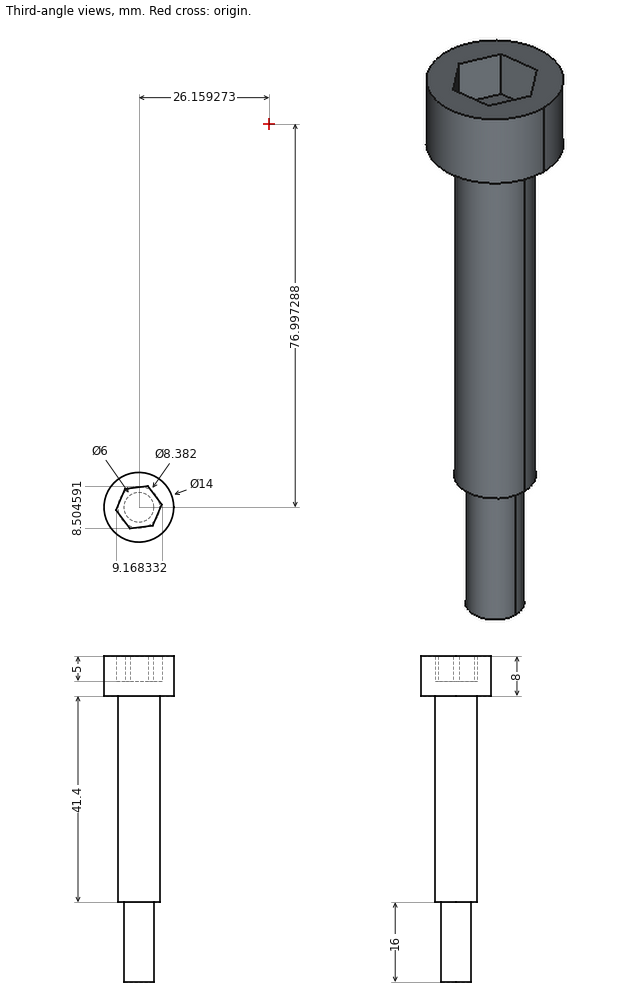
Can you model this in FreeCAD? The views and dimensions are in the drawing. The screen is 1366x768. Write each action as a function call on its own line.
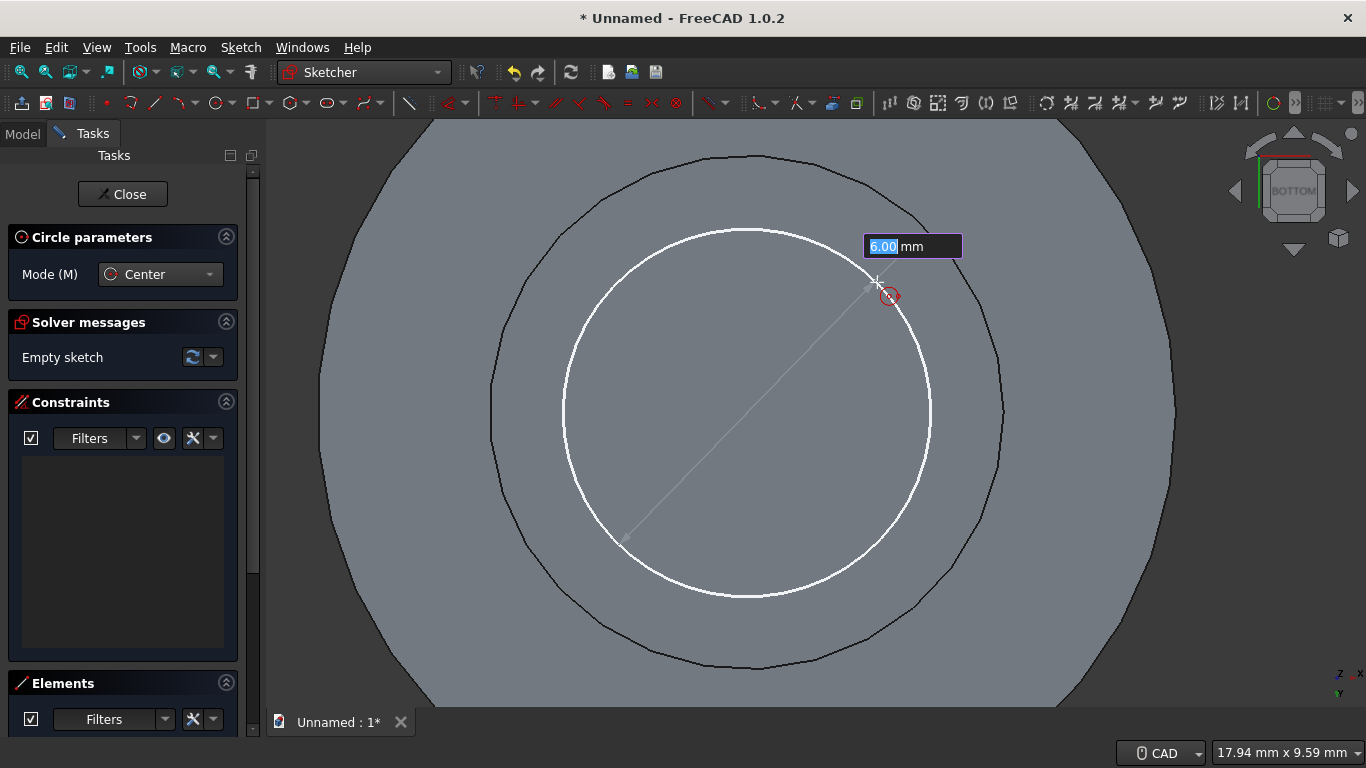
text(6)
key(Return)
key(Escape)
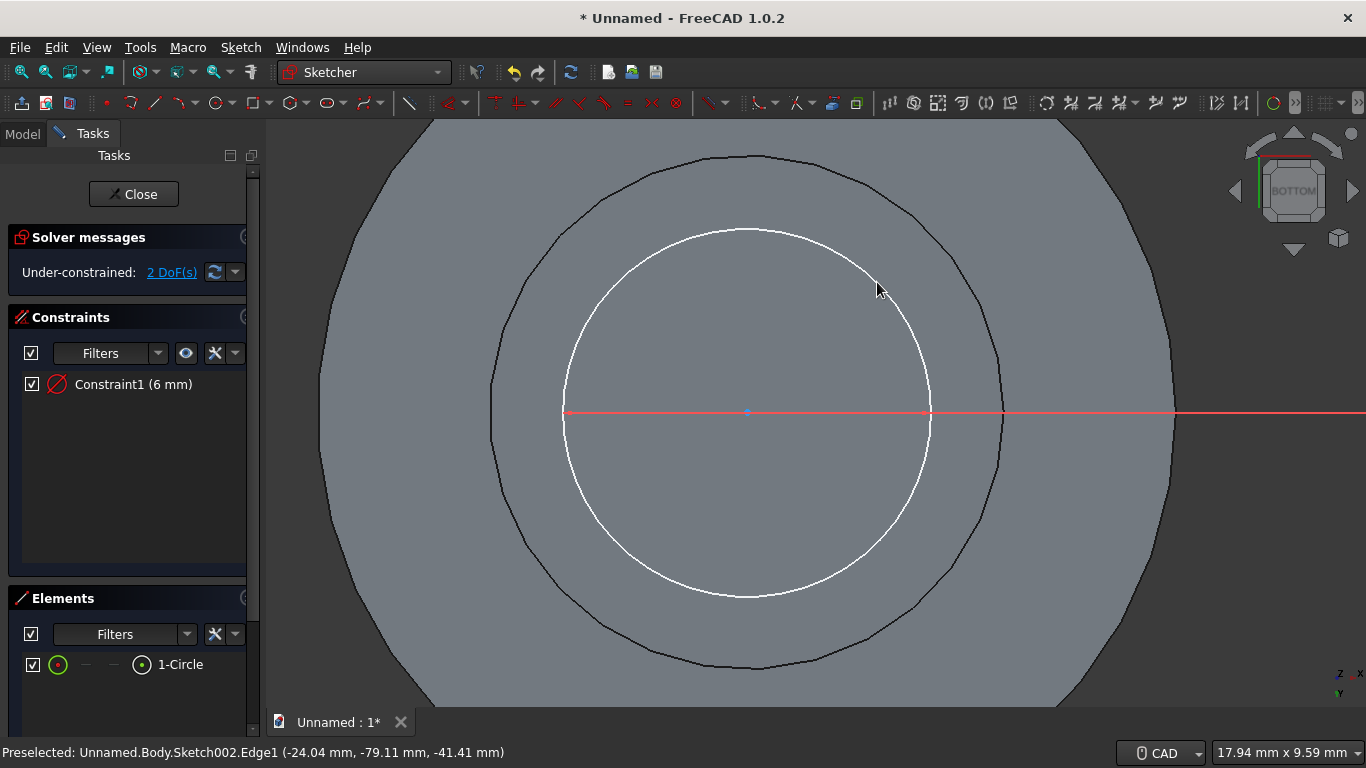
click(448, 104)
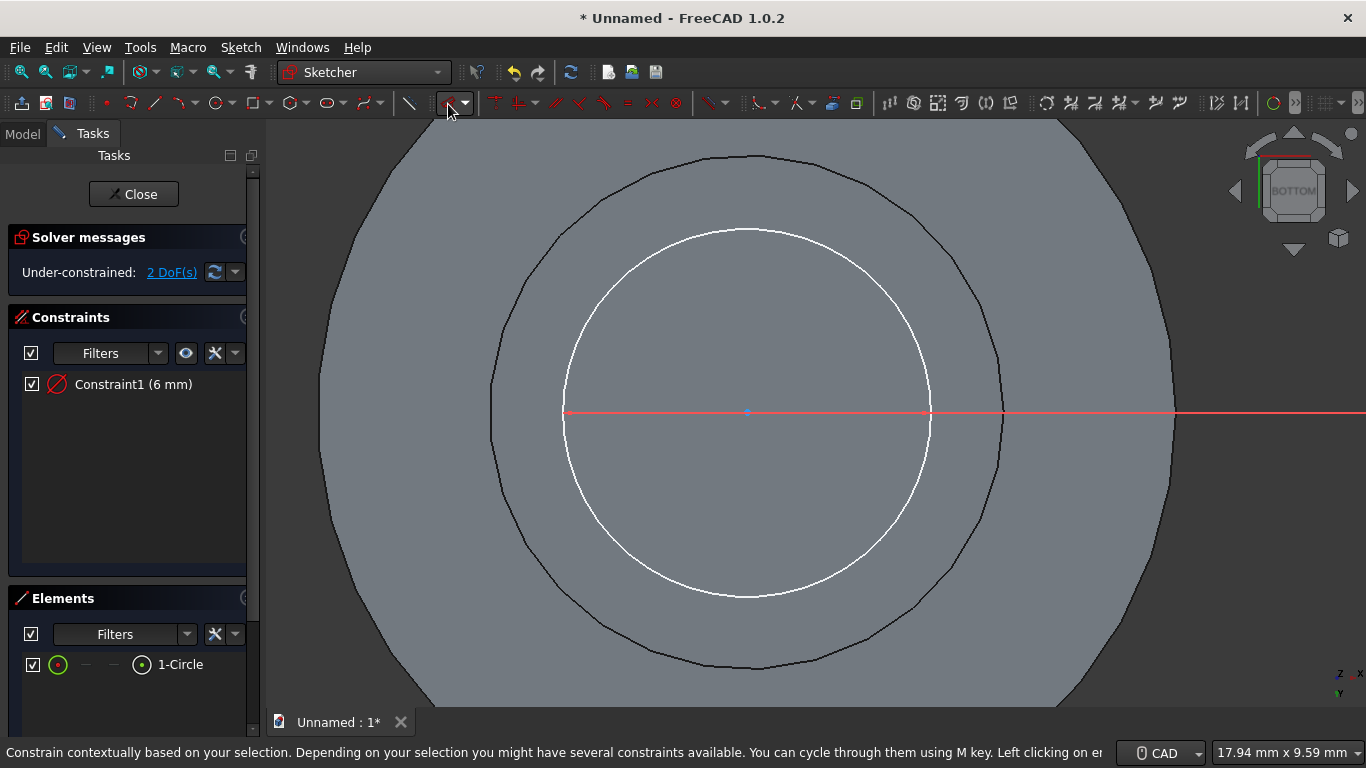
click(747, 413)
click(974, 379)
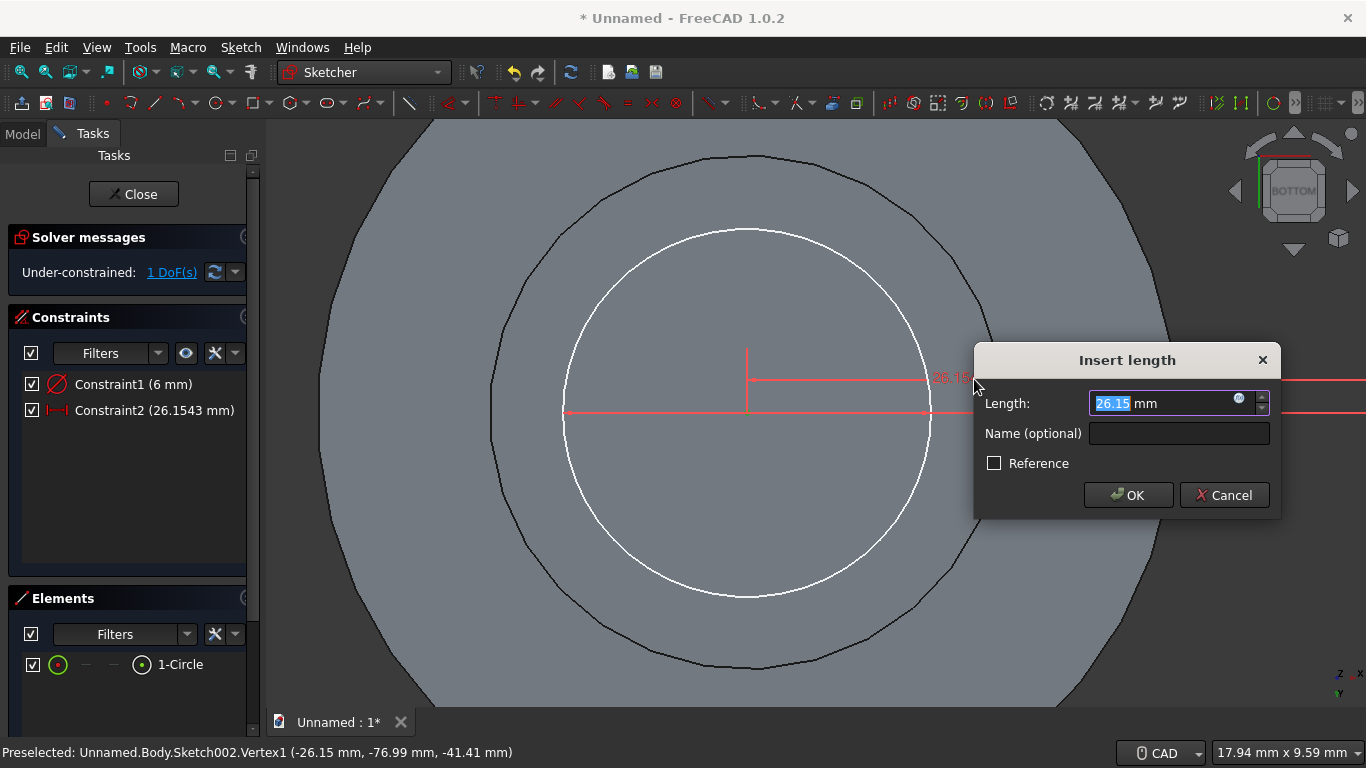
text(26.159273)
key(Return)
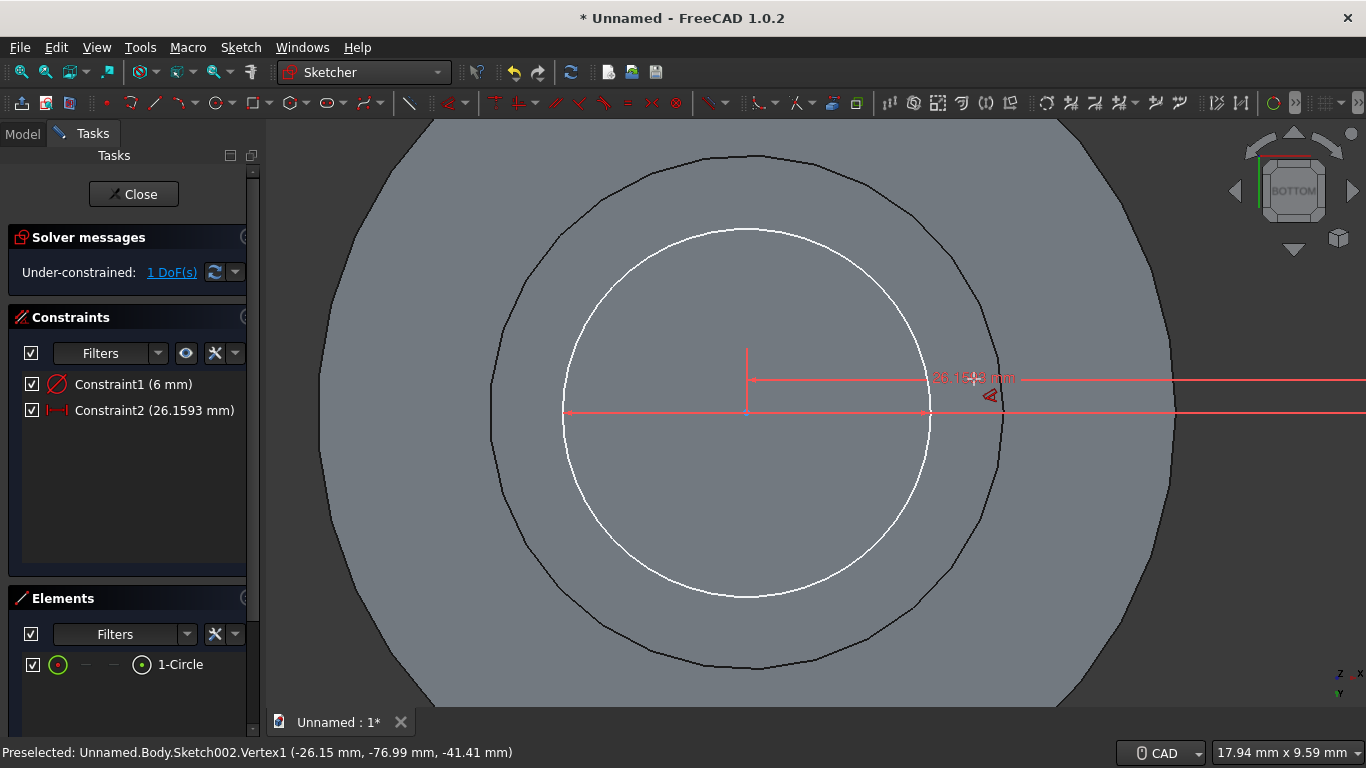
click(747, 413)
click(713, 546)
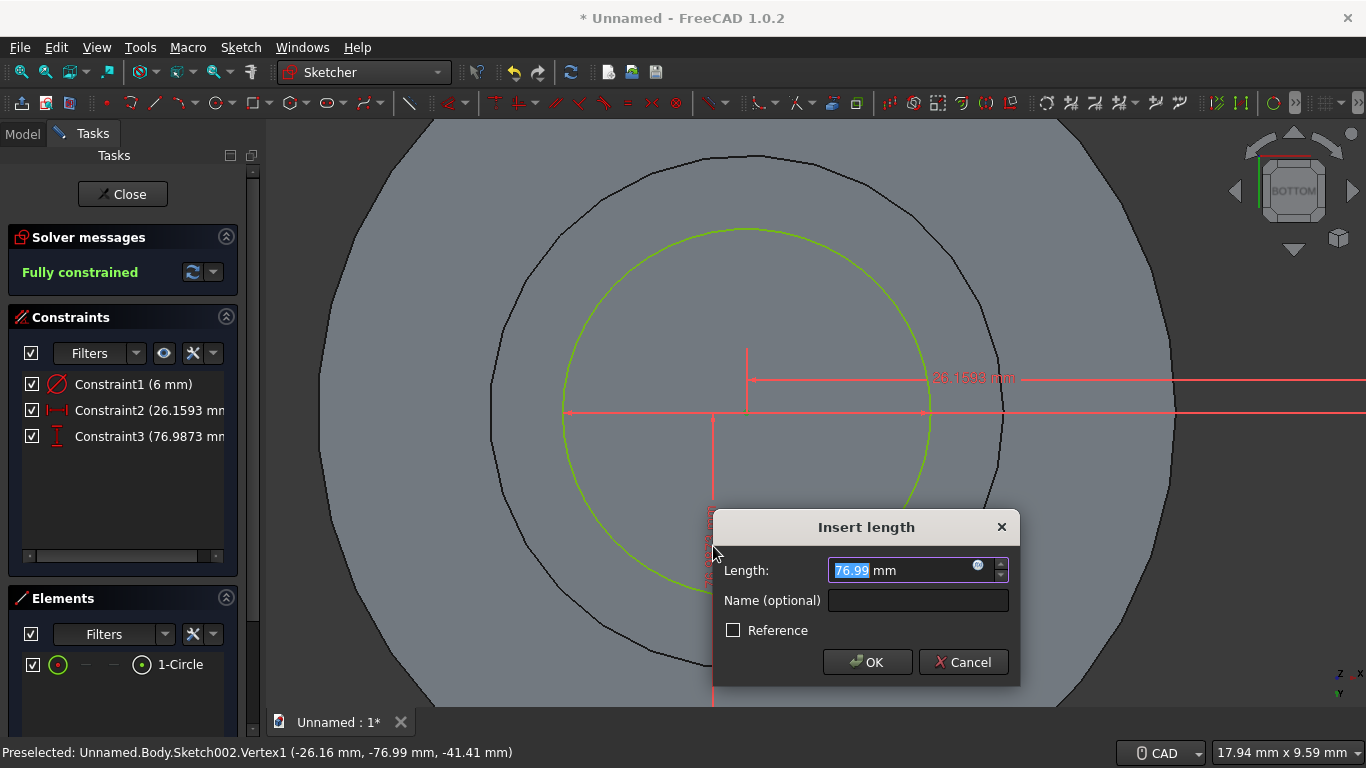
text(76.997288)
key(Return)
key(Escape)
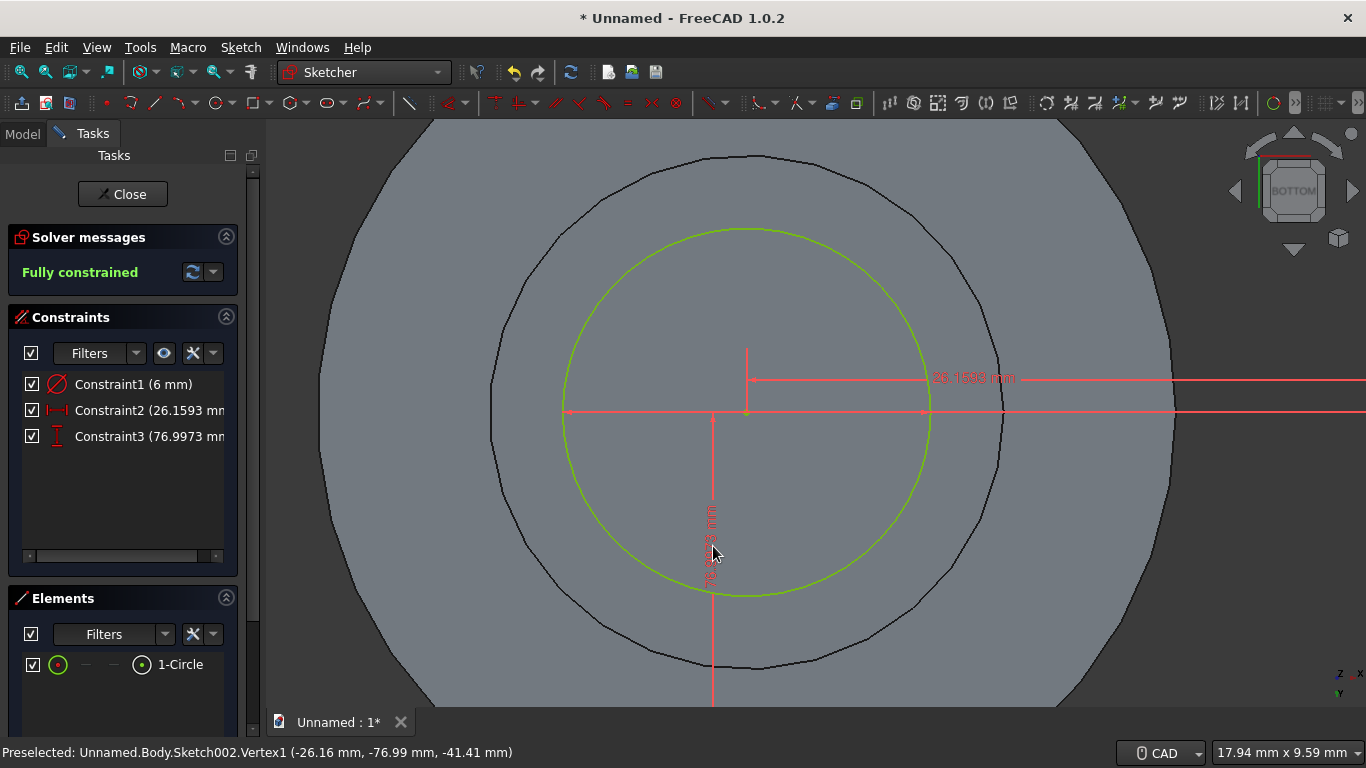
click(123, 194)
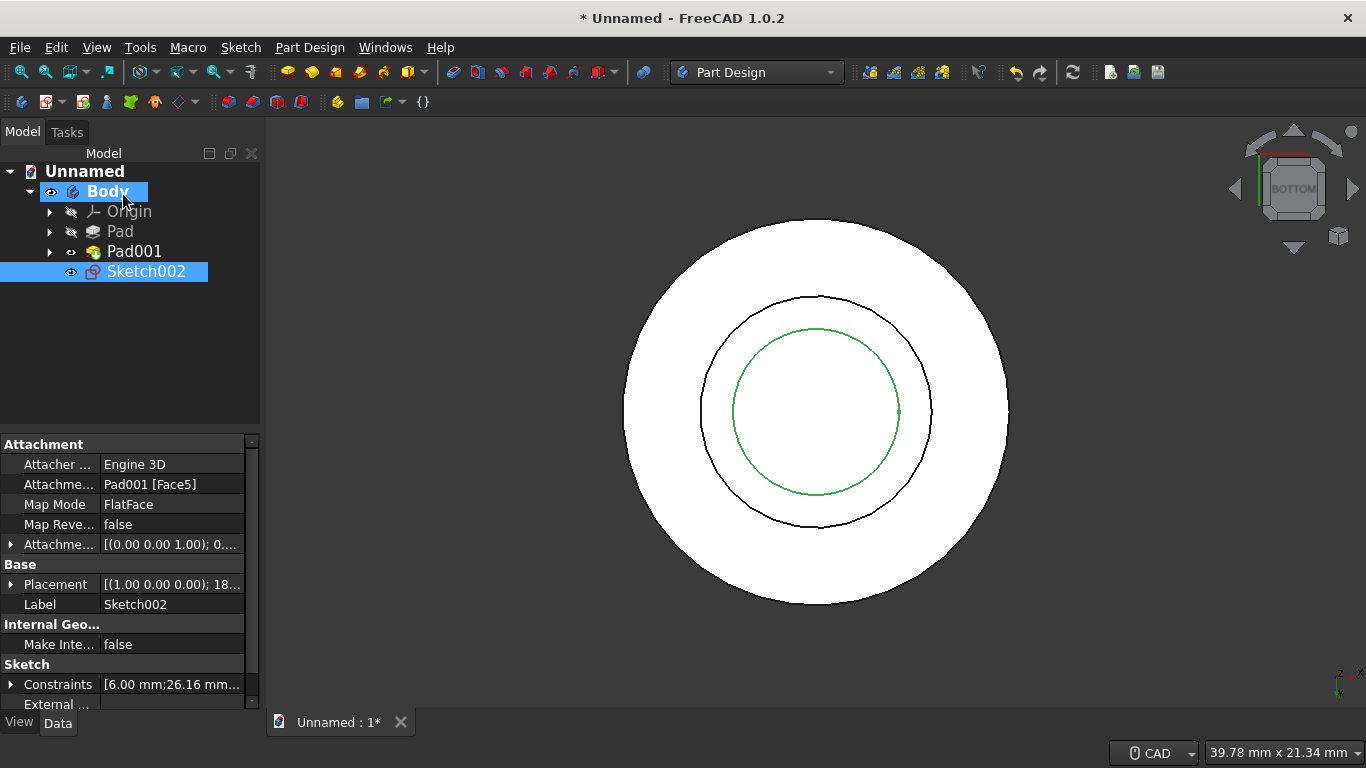
click(288, 72)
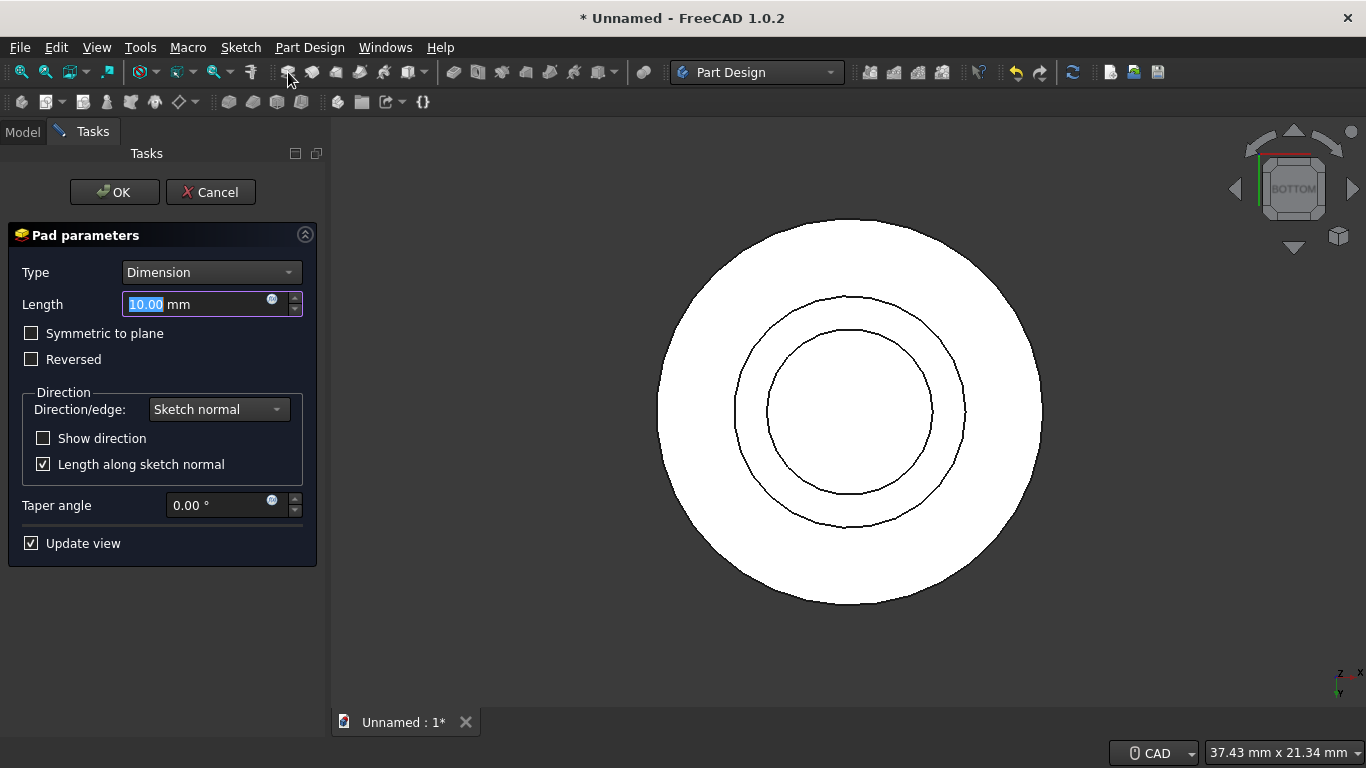
text(16)
key(Tab)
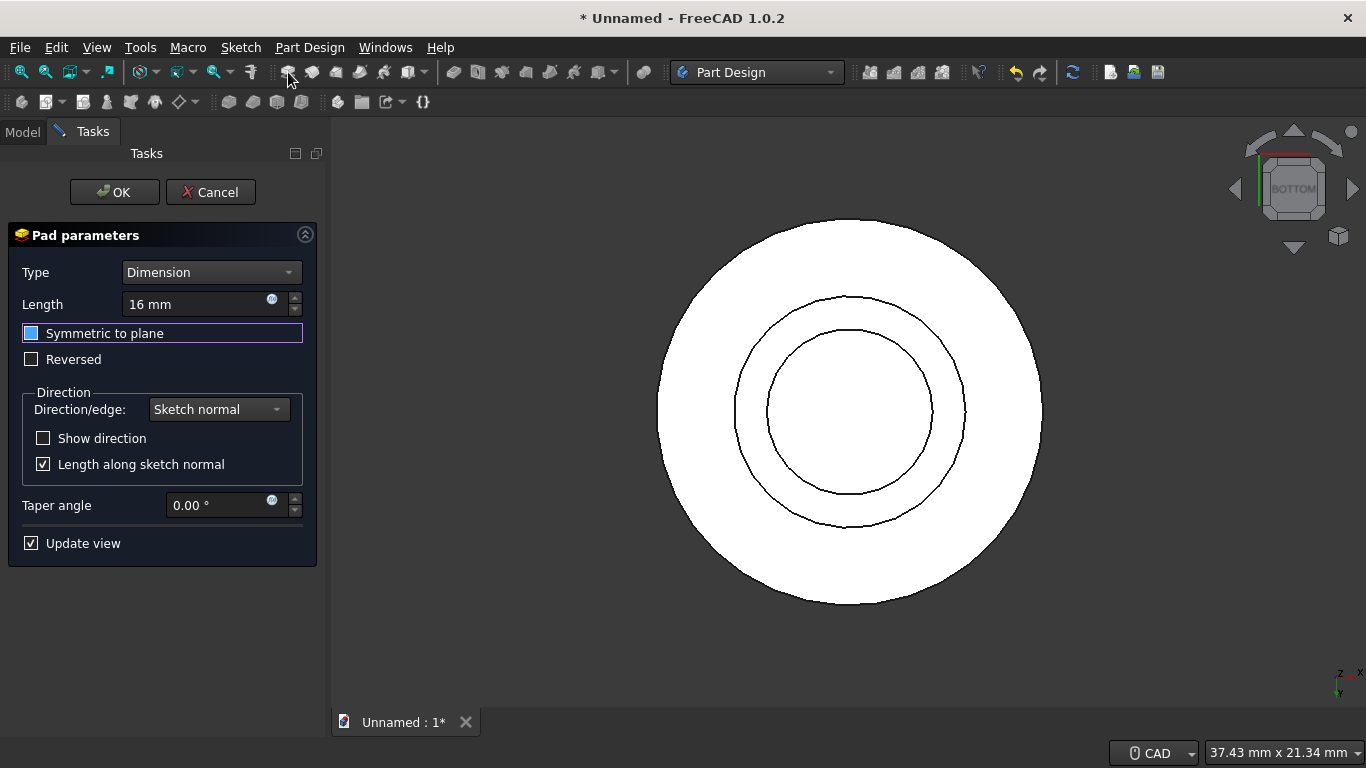
click(115, 192)